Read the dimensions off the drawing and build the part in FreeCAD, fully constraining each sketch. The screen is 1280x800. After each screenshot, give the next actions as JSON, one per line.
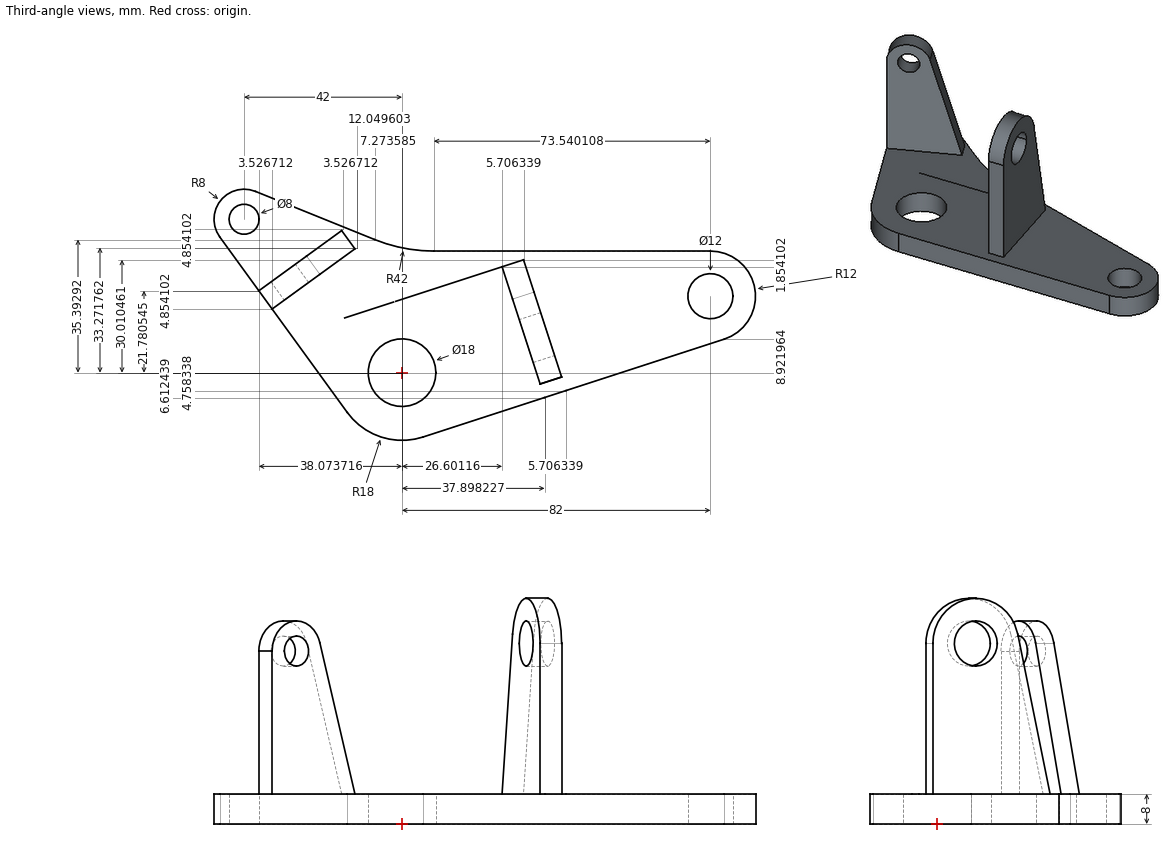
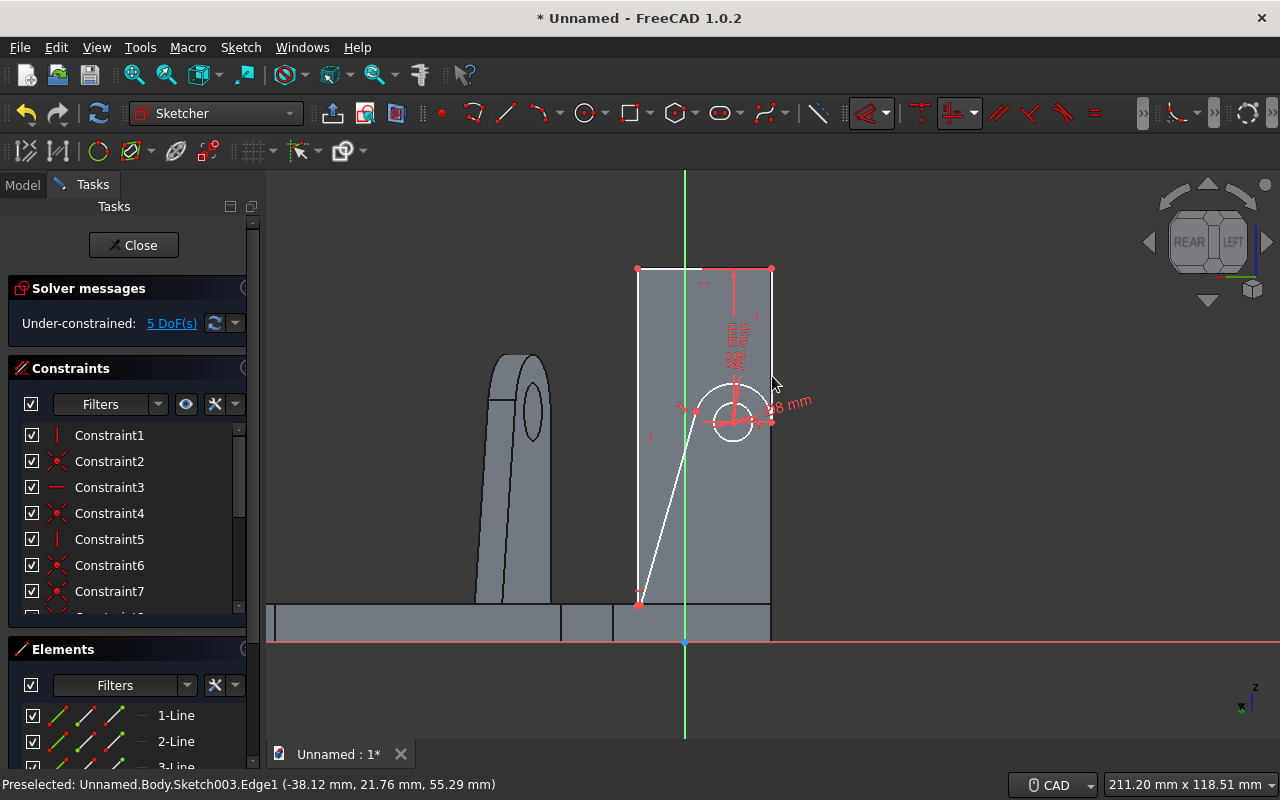
{"action": "left_click", "coordinate": [638, 370]}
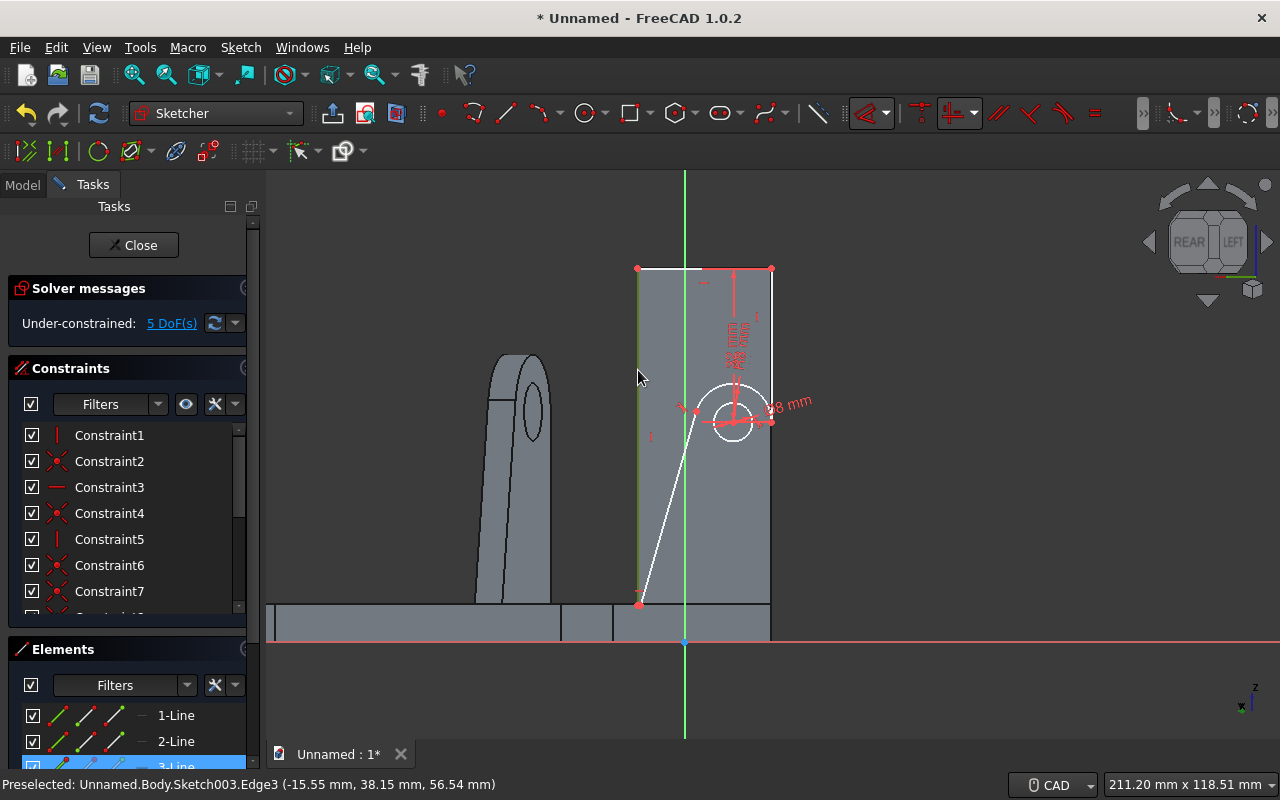
{"action": "left_click", "coordinate": [888, 114]}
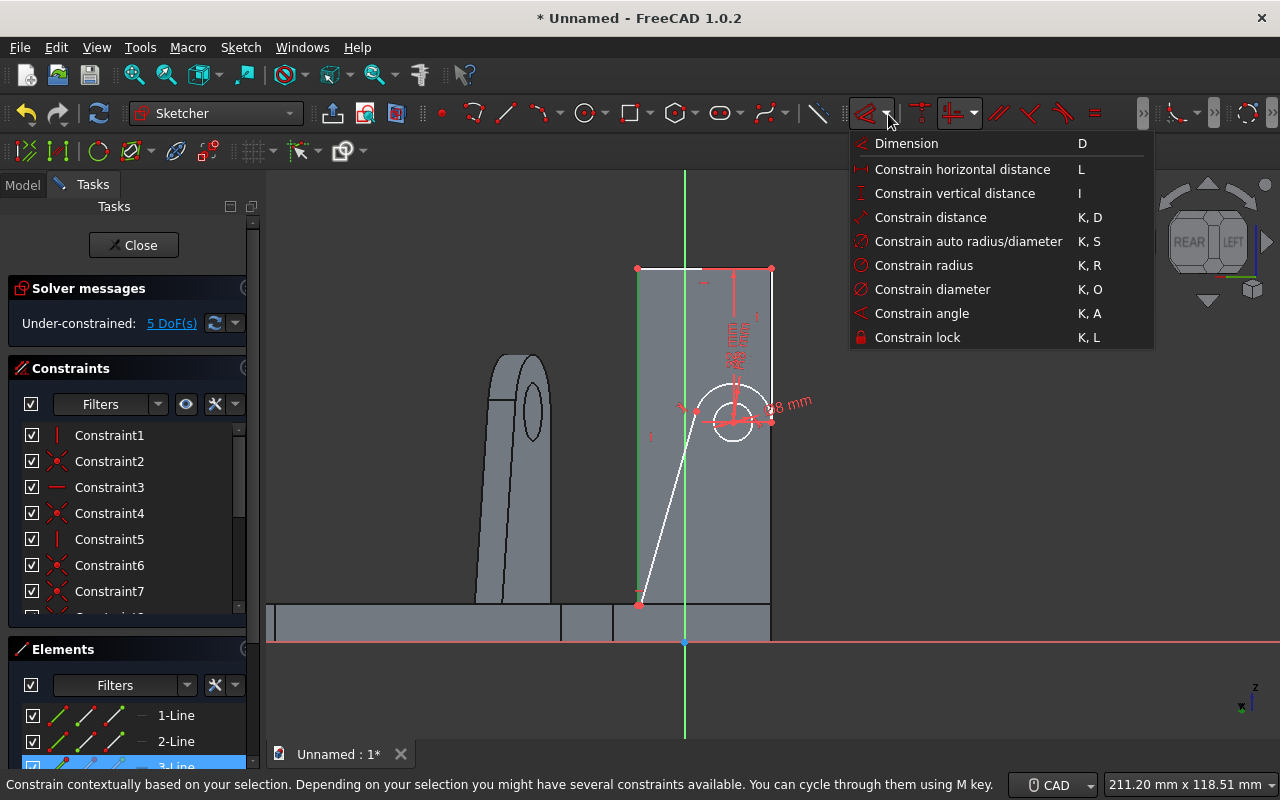
{"action": "left_click", "coordinate": [1002, 193]}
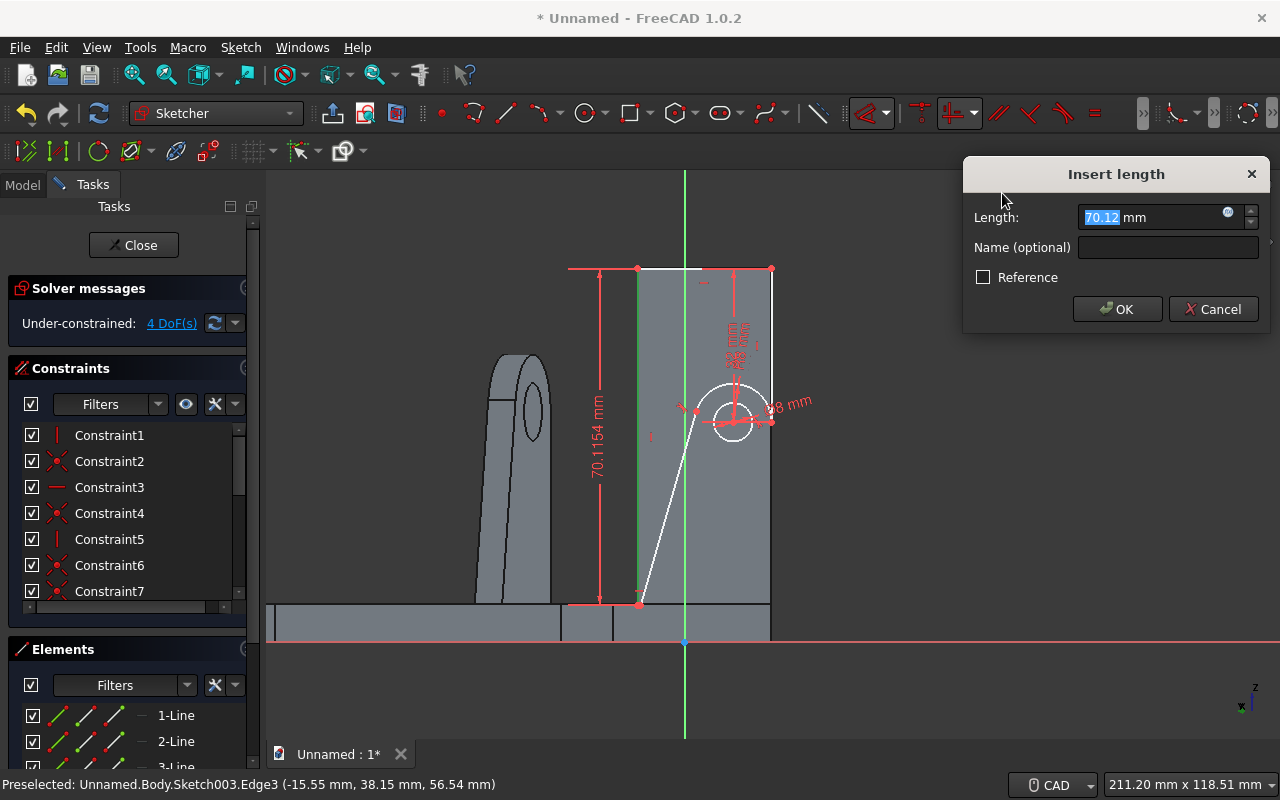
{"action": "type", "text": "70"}
{"action": "key", "text": "Return"}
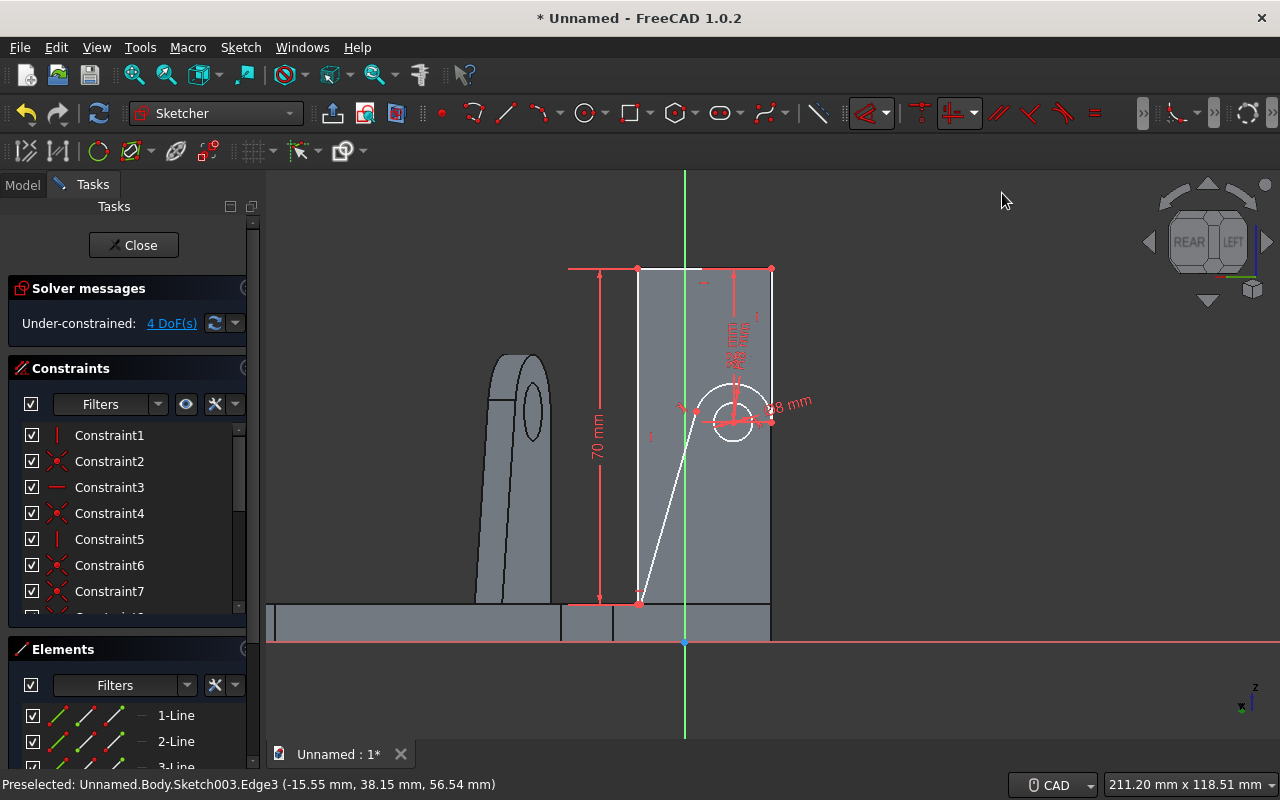
{"action": "scroll", "coordinate": [638, 605], "scroll_direction": "up", "scroll_amount": 7}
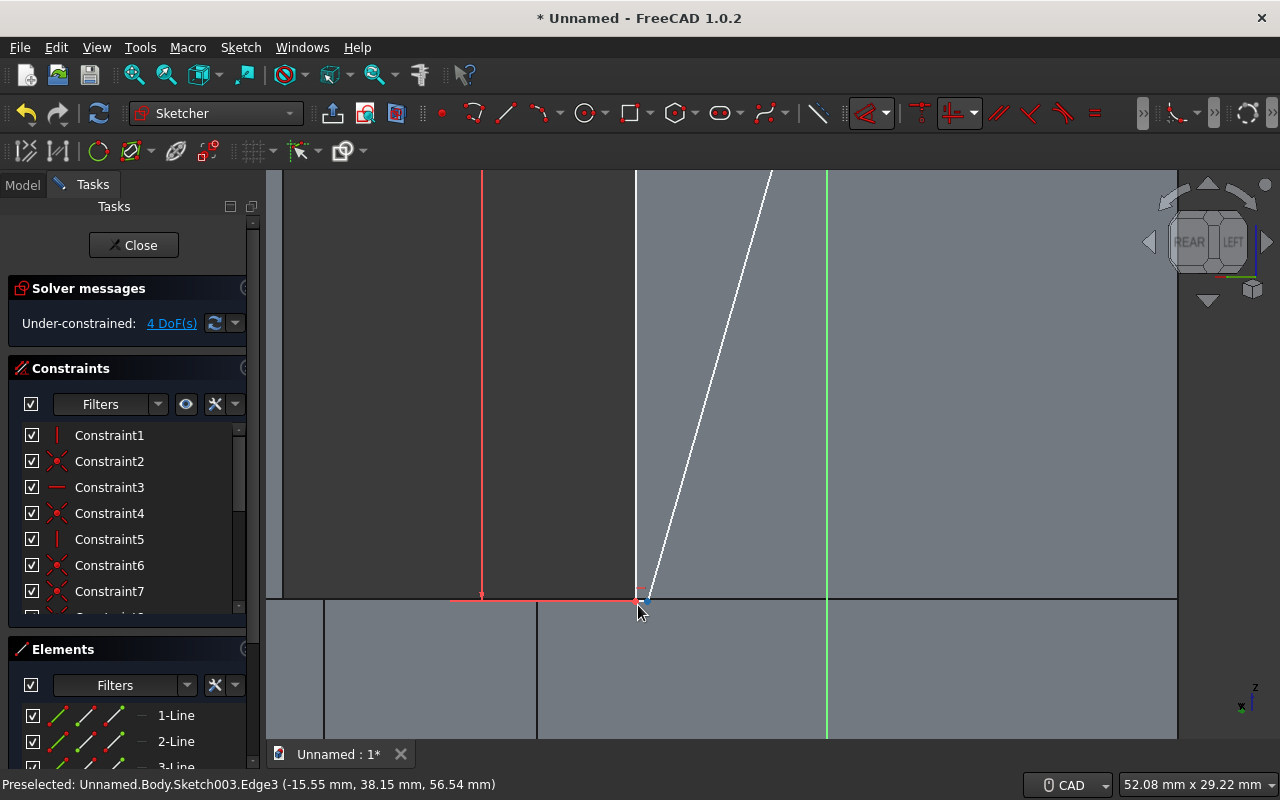
{"action": "left_click", "coordinate": [636, 601]}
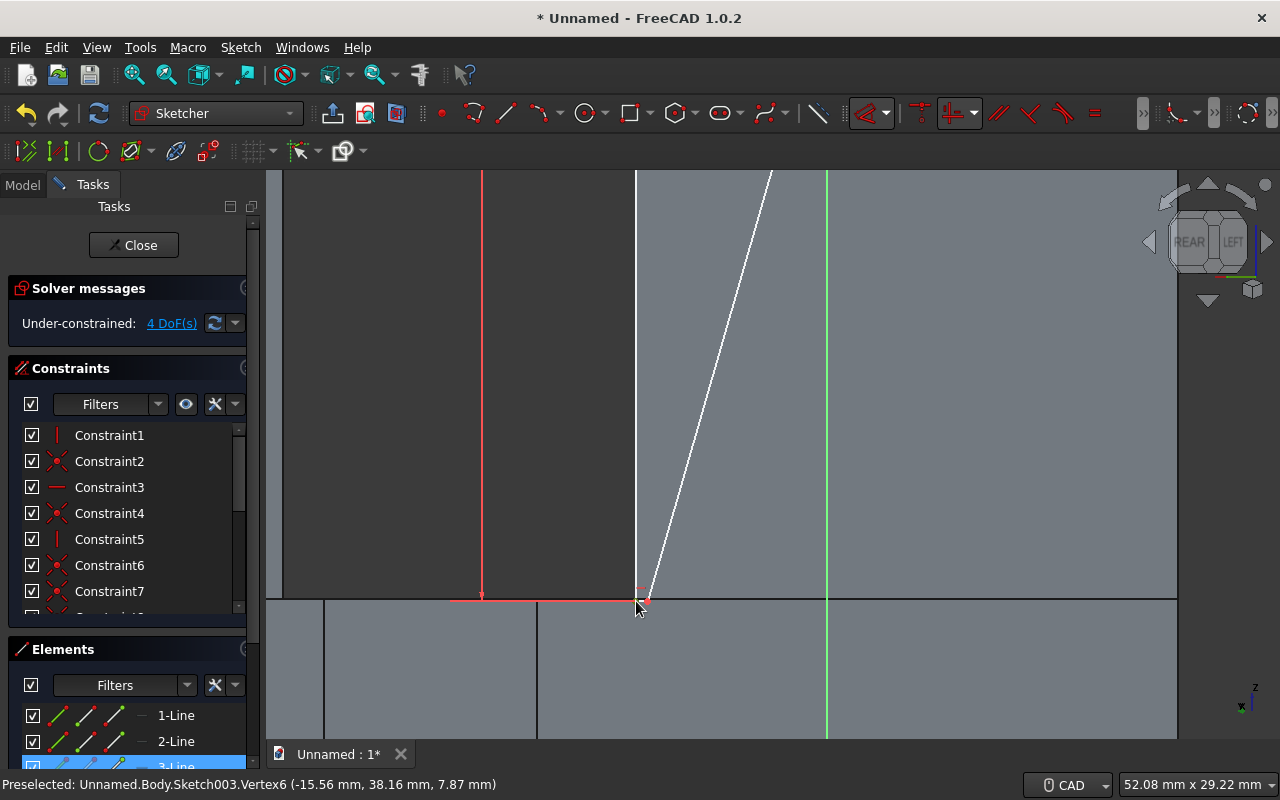
{"action": "key", "text": "i"}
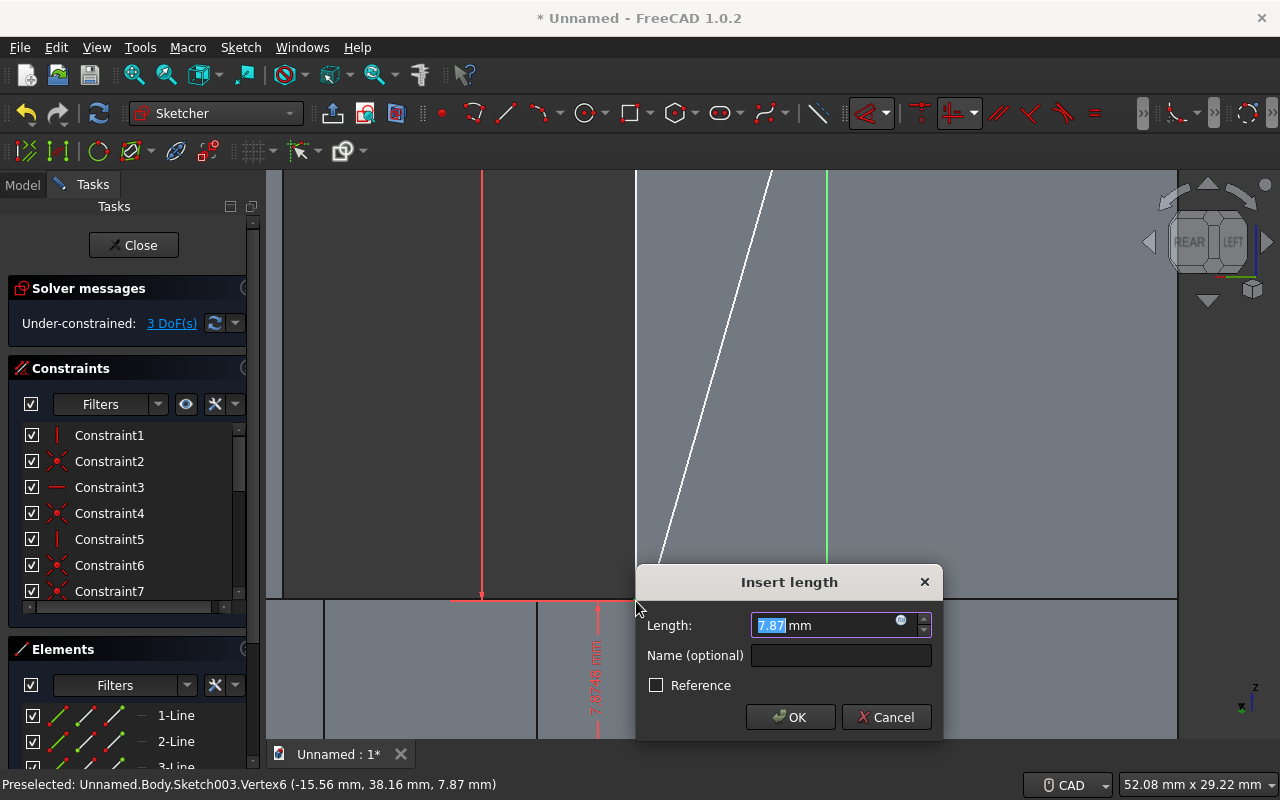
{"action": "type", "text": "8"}
{"action": "key", "text": "Return"}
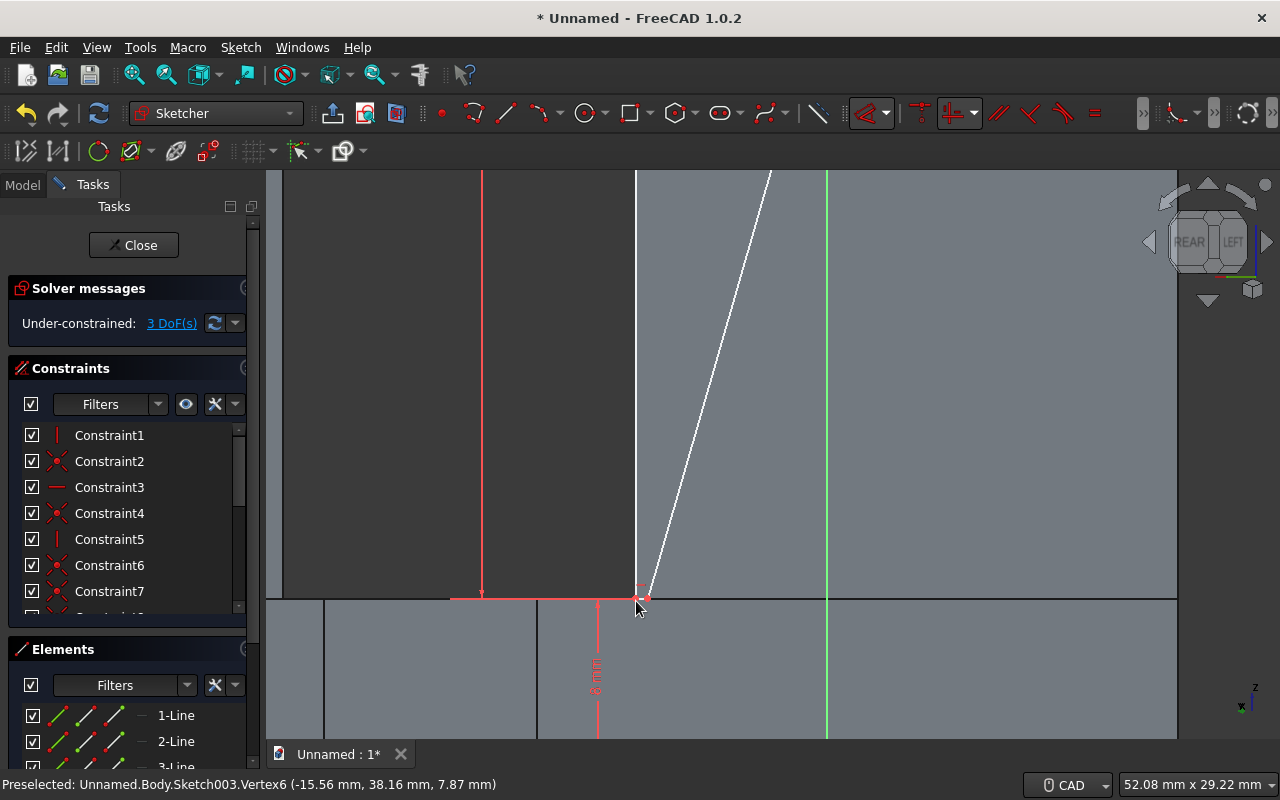
{"action": "scroll", "coordinate": [638, 605], "scroll_direction": "down", "scroll_amount": 7}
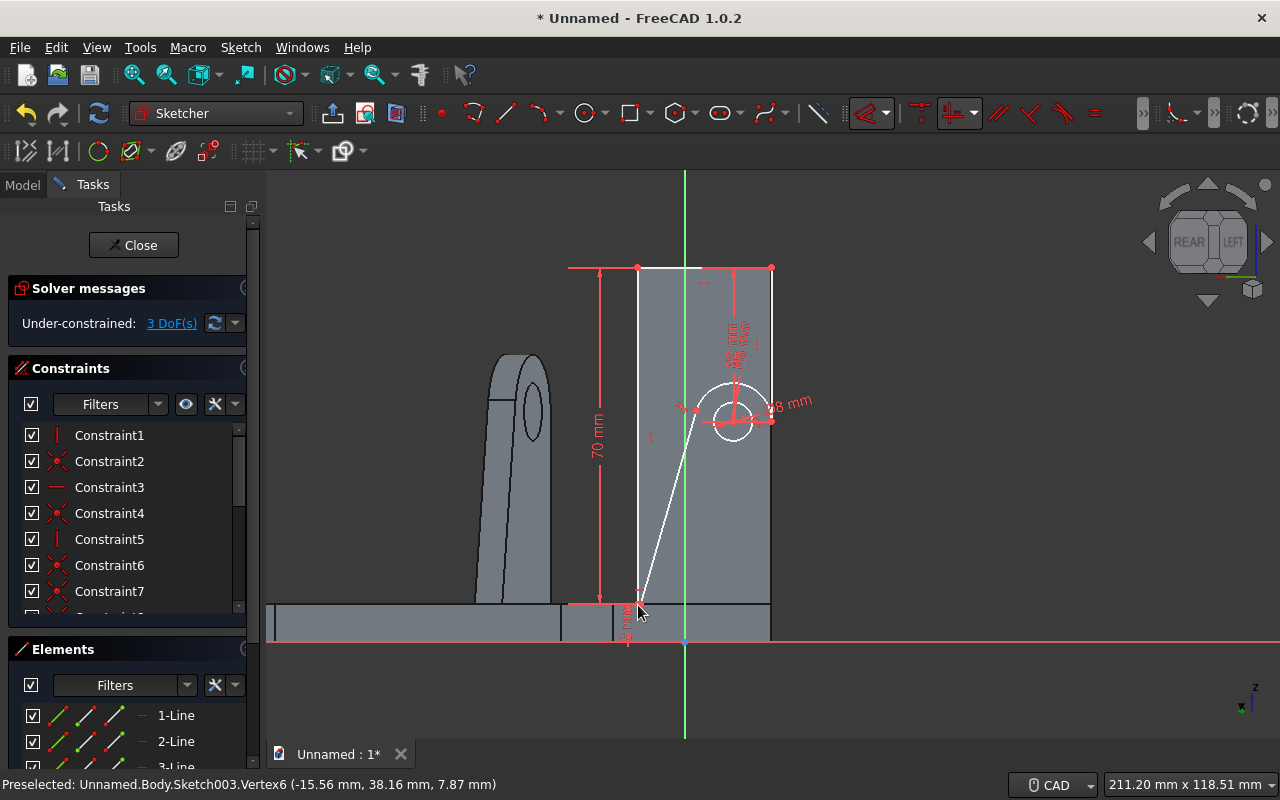
{"action": "left_click", "coordinate": [733, 422]}